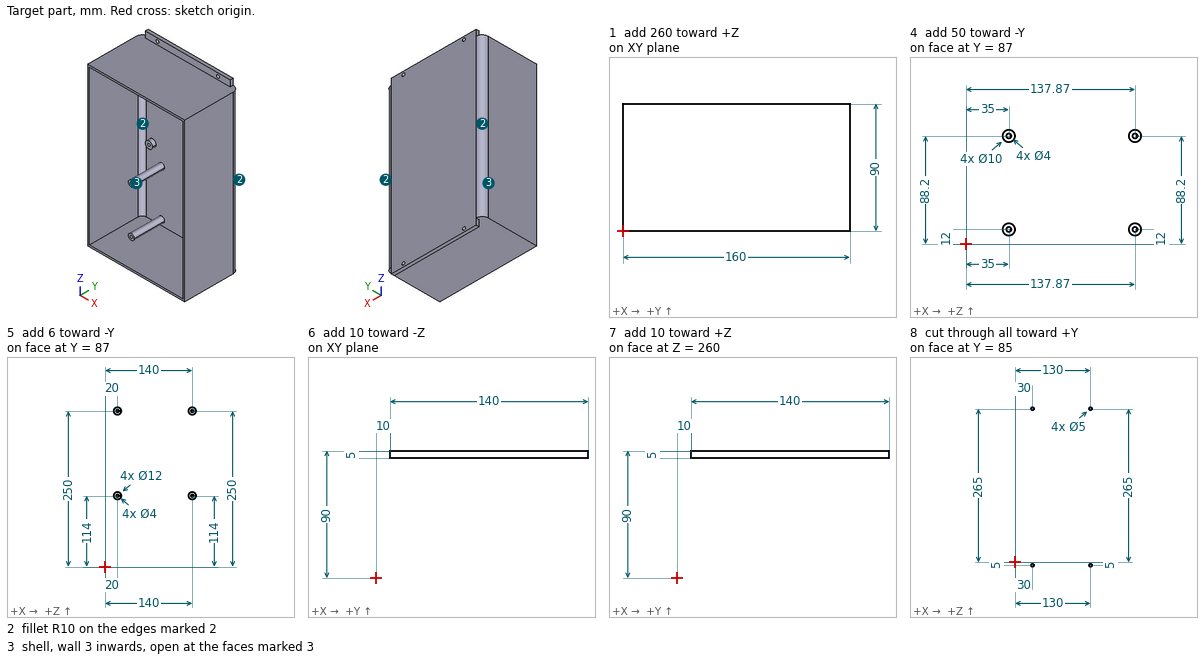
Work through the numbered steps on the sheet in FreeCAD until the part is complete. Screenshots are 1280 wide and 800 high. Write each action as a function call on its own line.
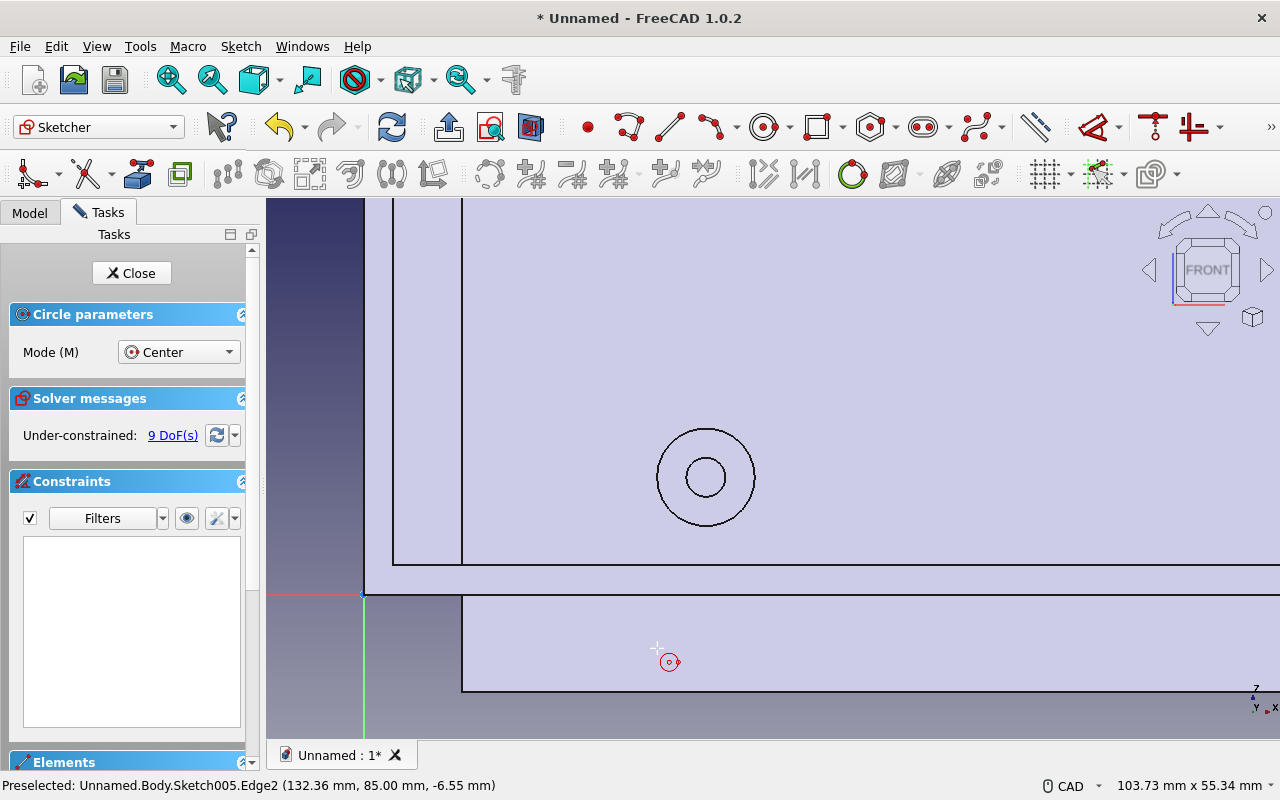
scroll(656, 648, down, 10)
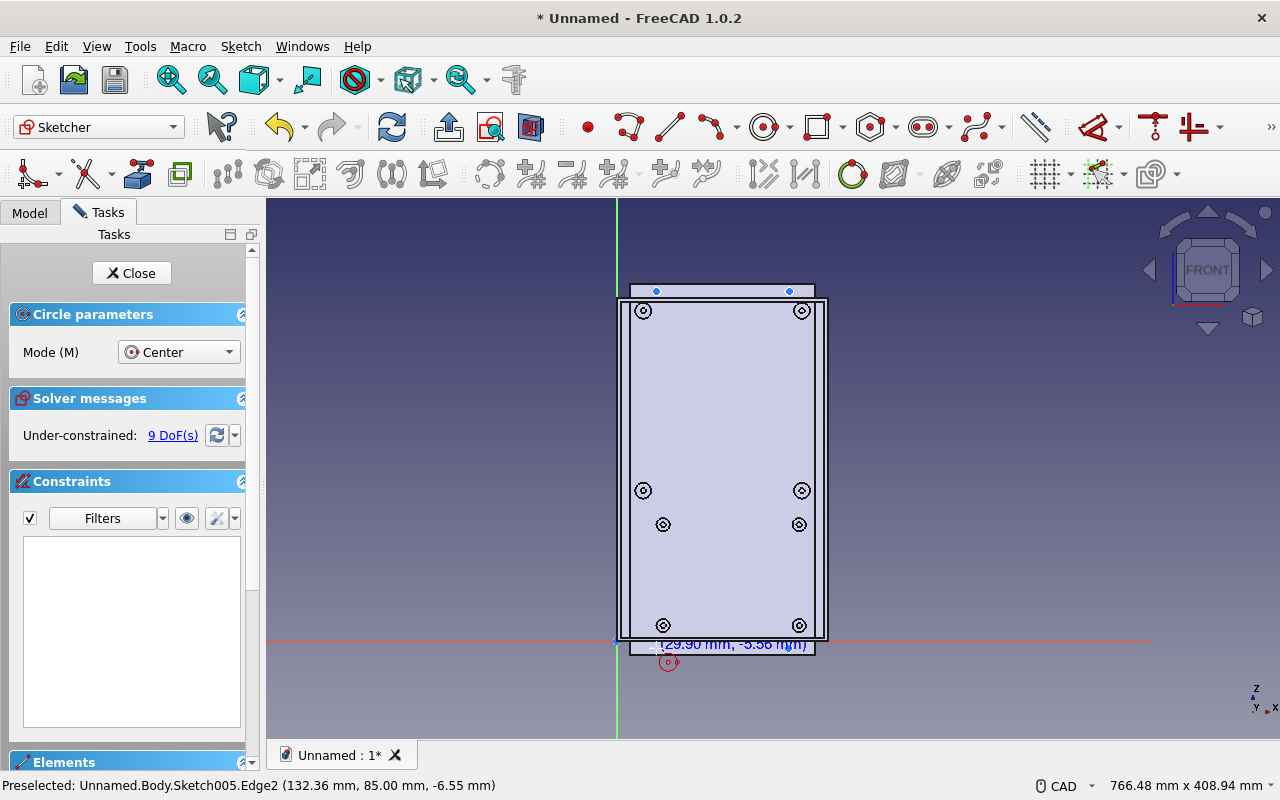
scroll(656, 648, up, 5)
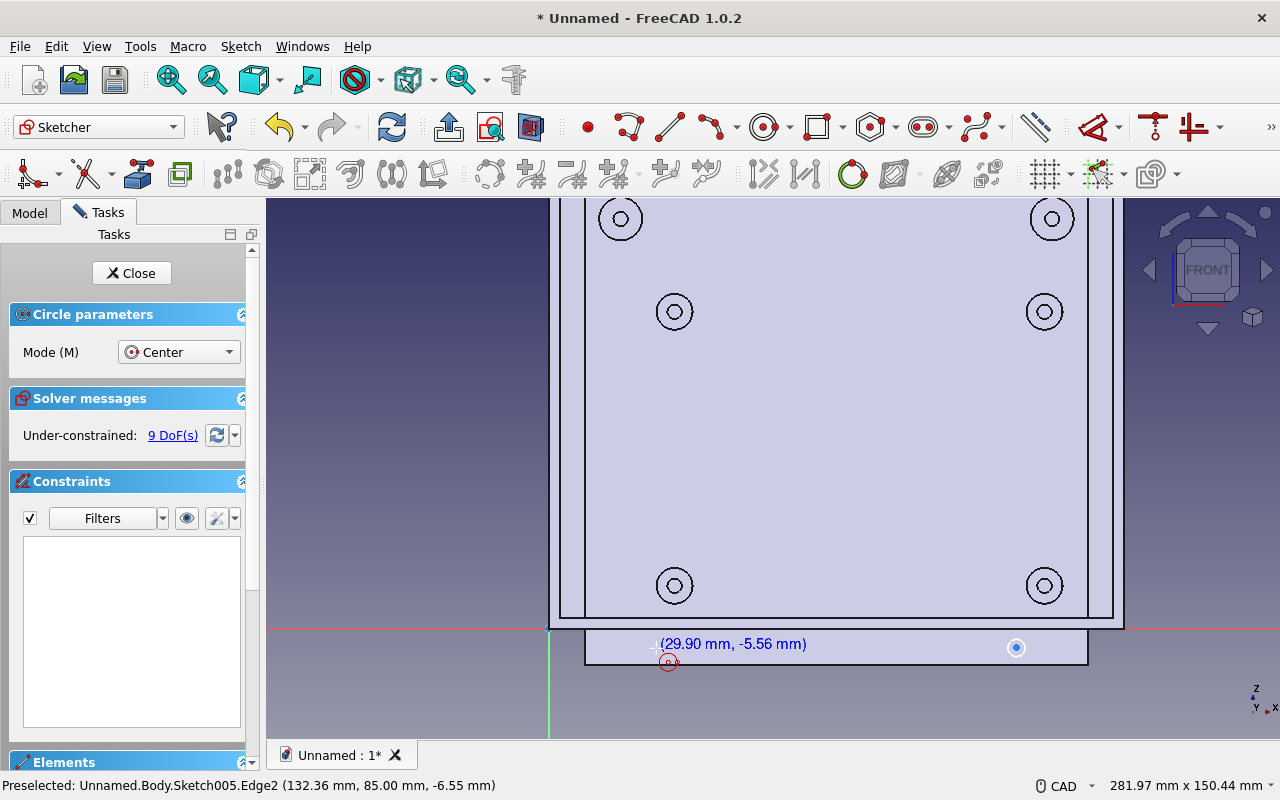
click(657, 647)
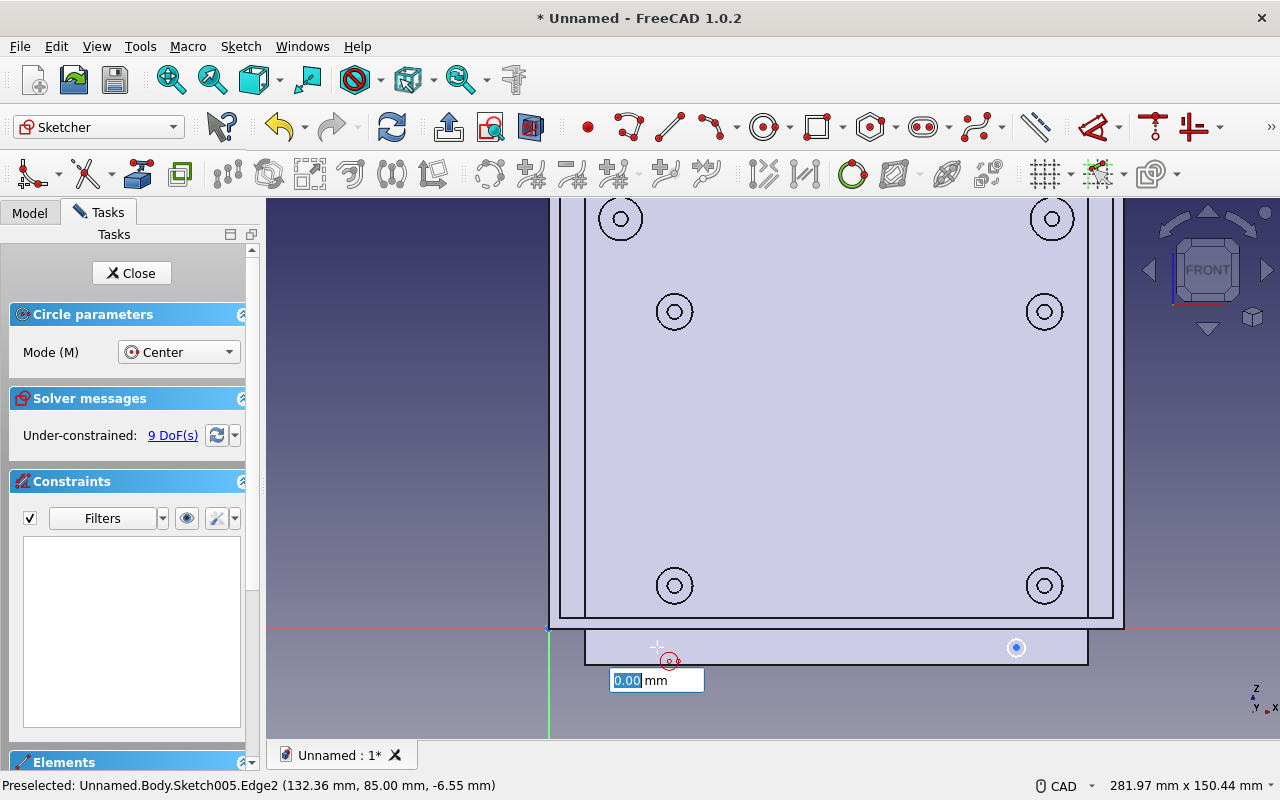
scroll(663, 653, up, 3)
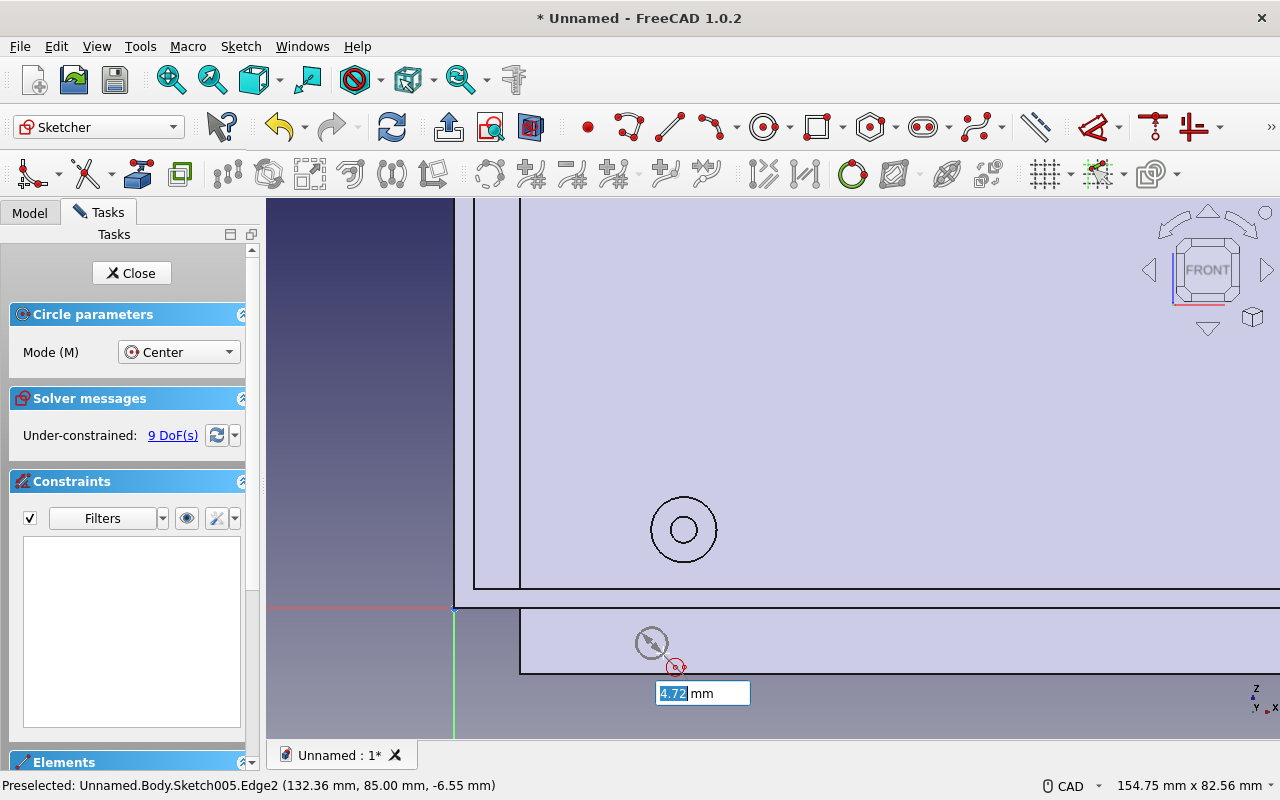
click(663, 653)
key(Escape)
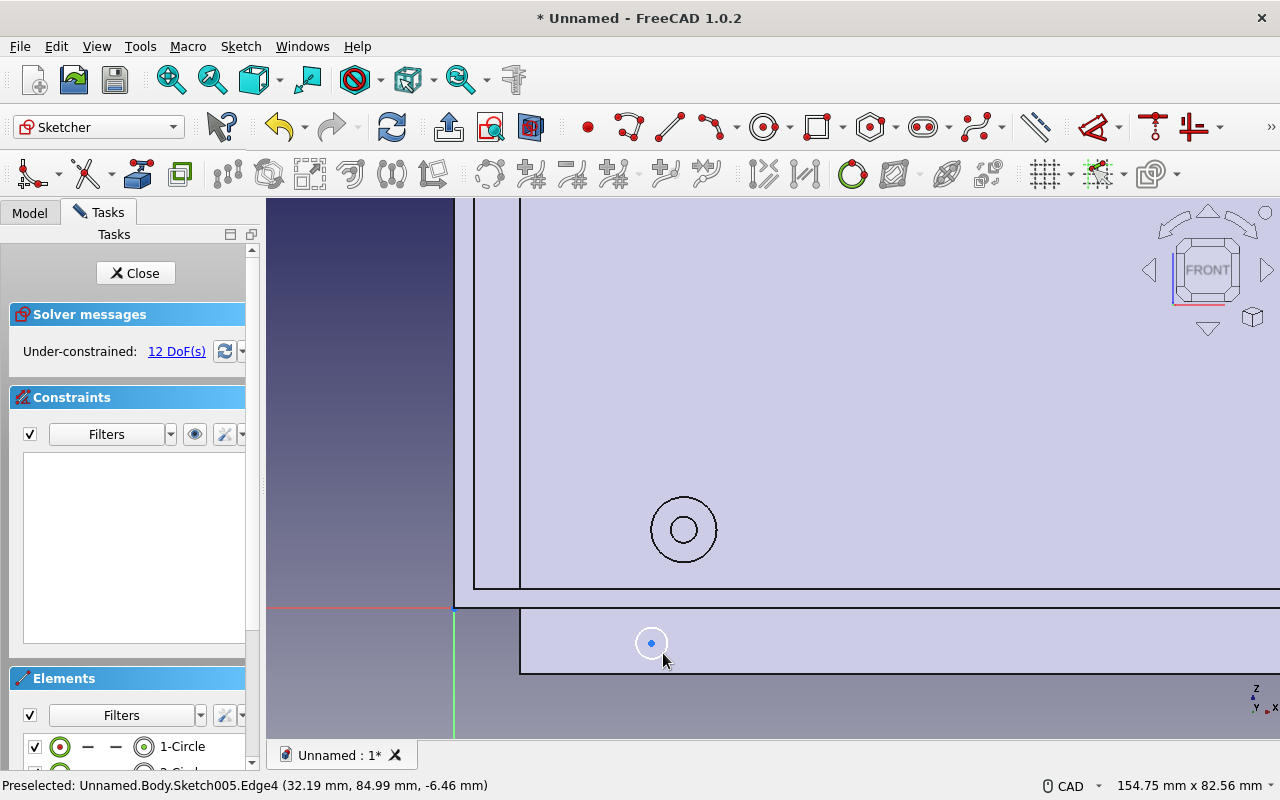
scroll(658, 649, down, 8)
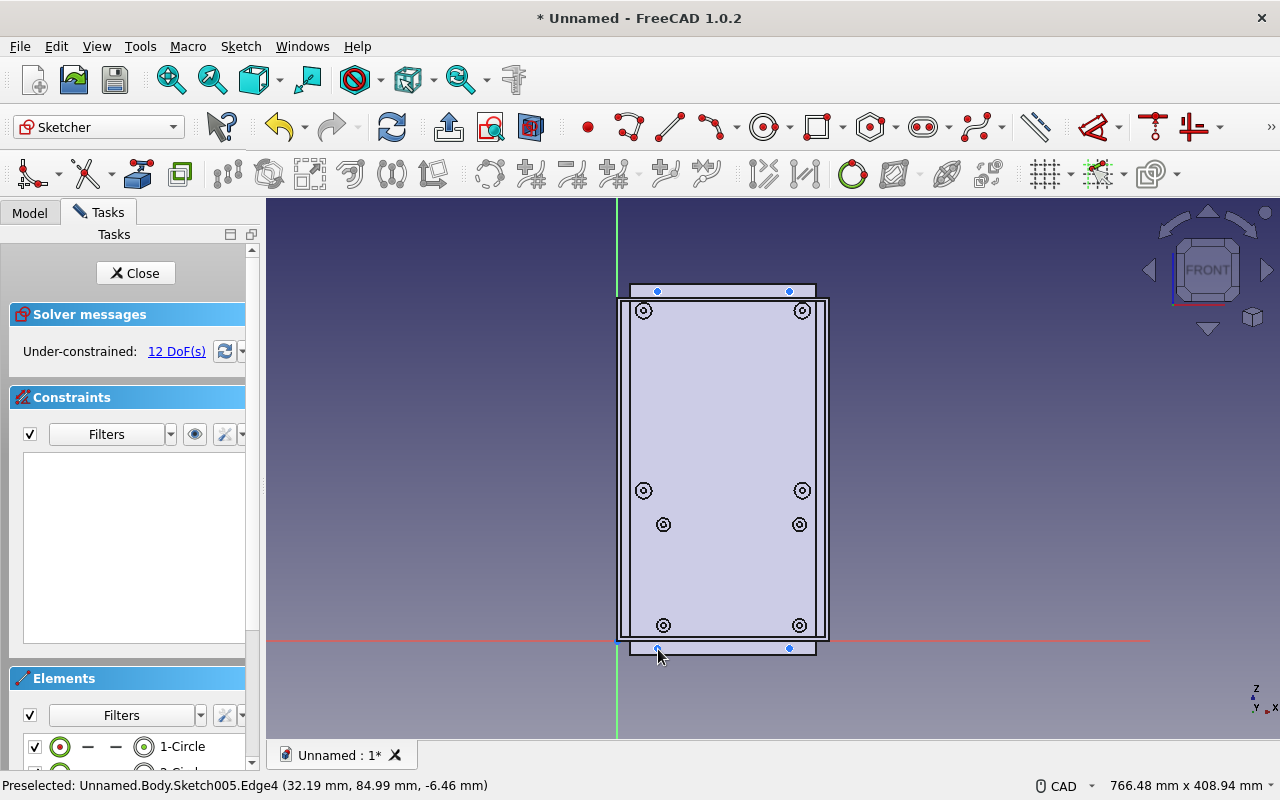
scroll(792, 289, up, 7)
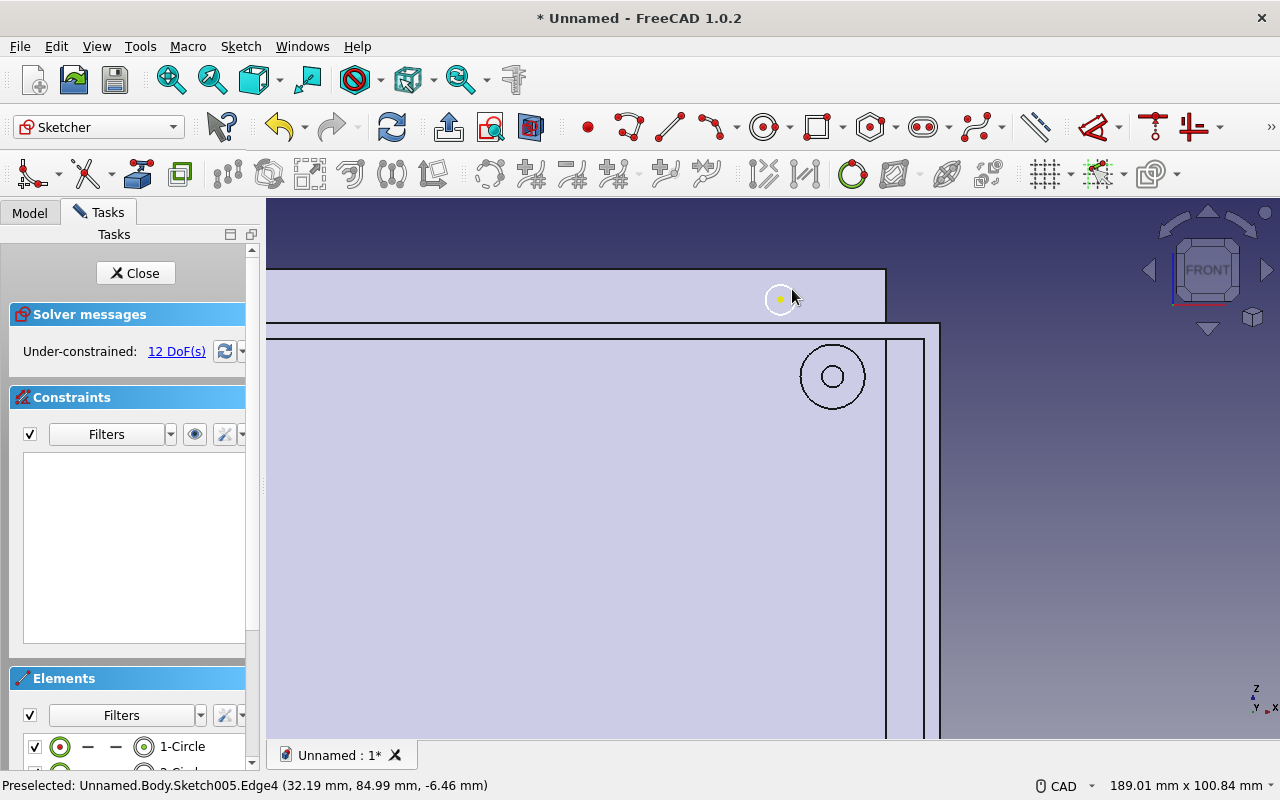
click(791, 289)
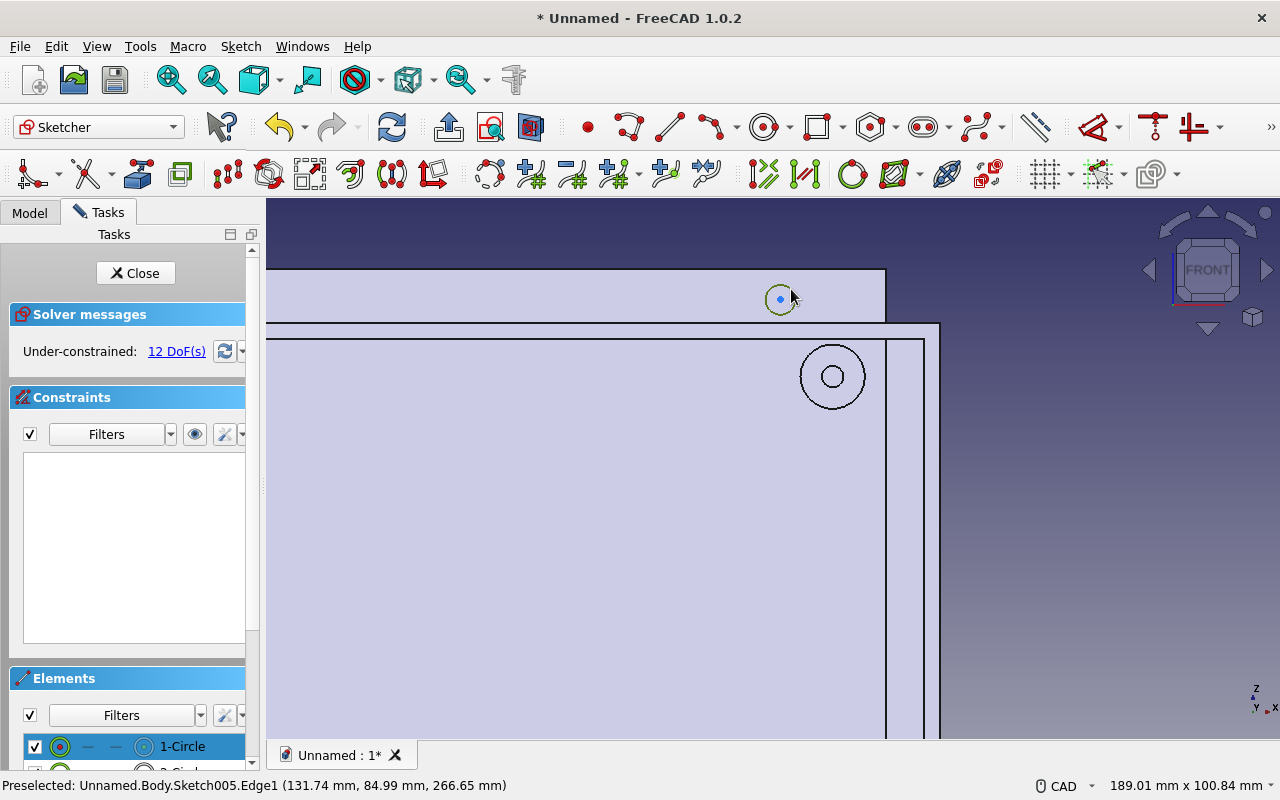
scroll(792, 288, down, 7)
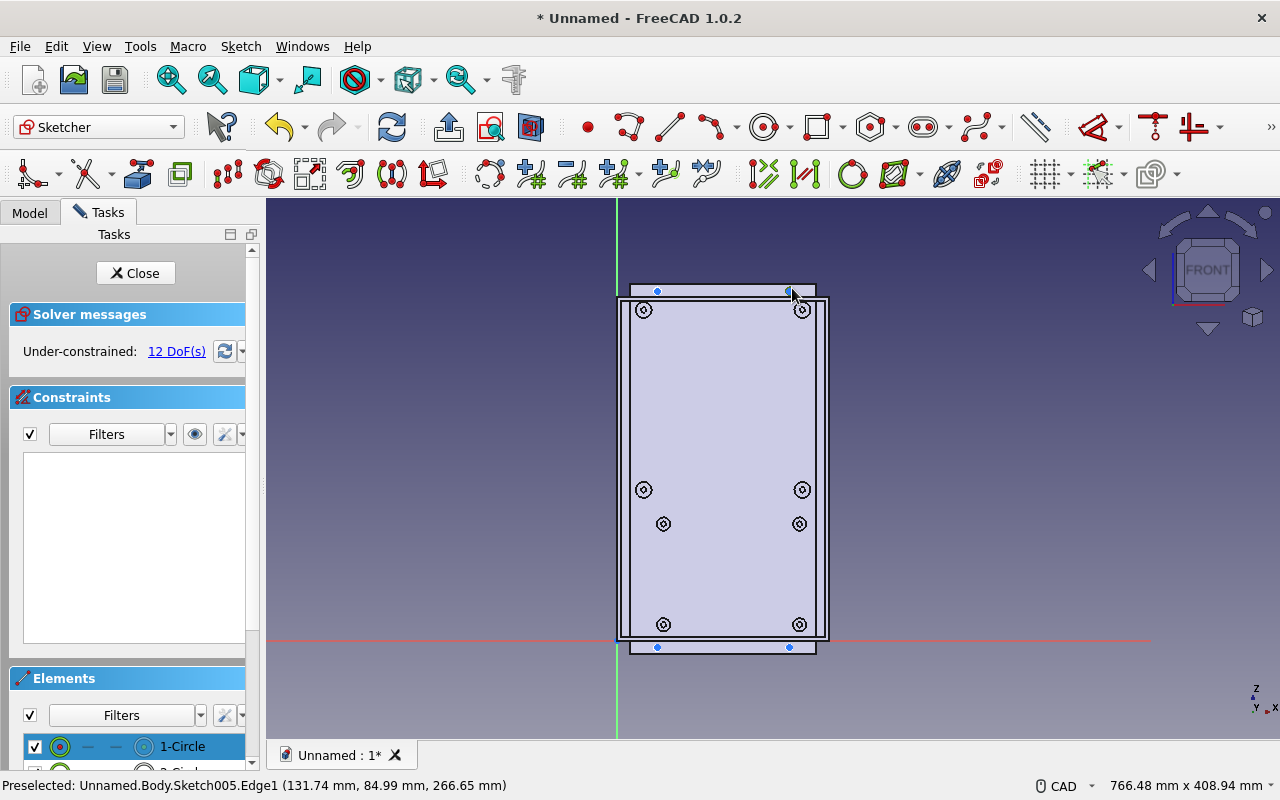
scroll(660, 288, up, 7)